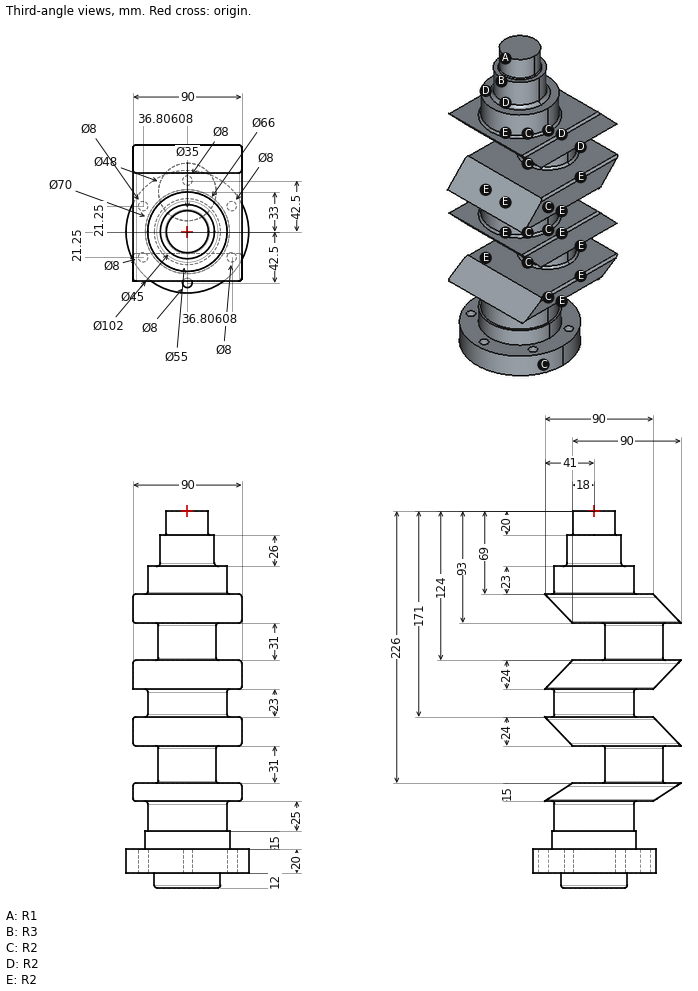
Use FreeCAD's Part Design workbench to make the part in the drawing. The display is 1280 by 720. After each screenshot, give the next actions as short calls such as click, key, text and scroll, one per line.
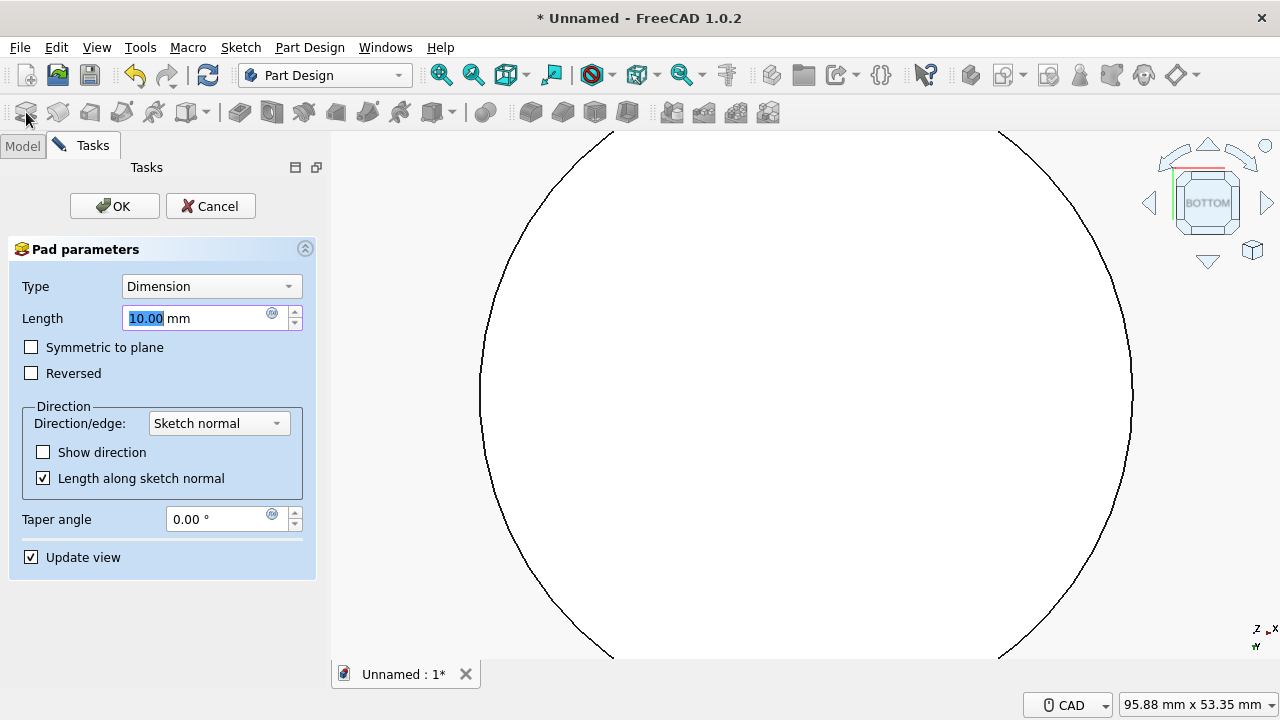
text(23)
key(Tab)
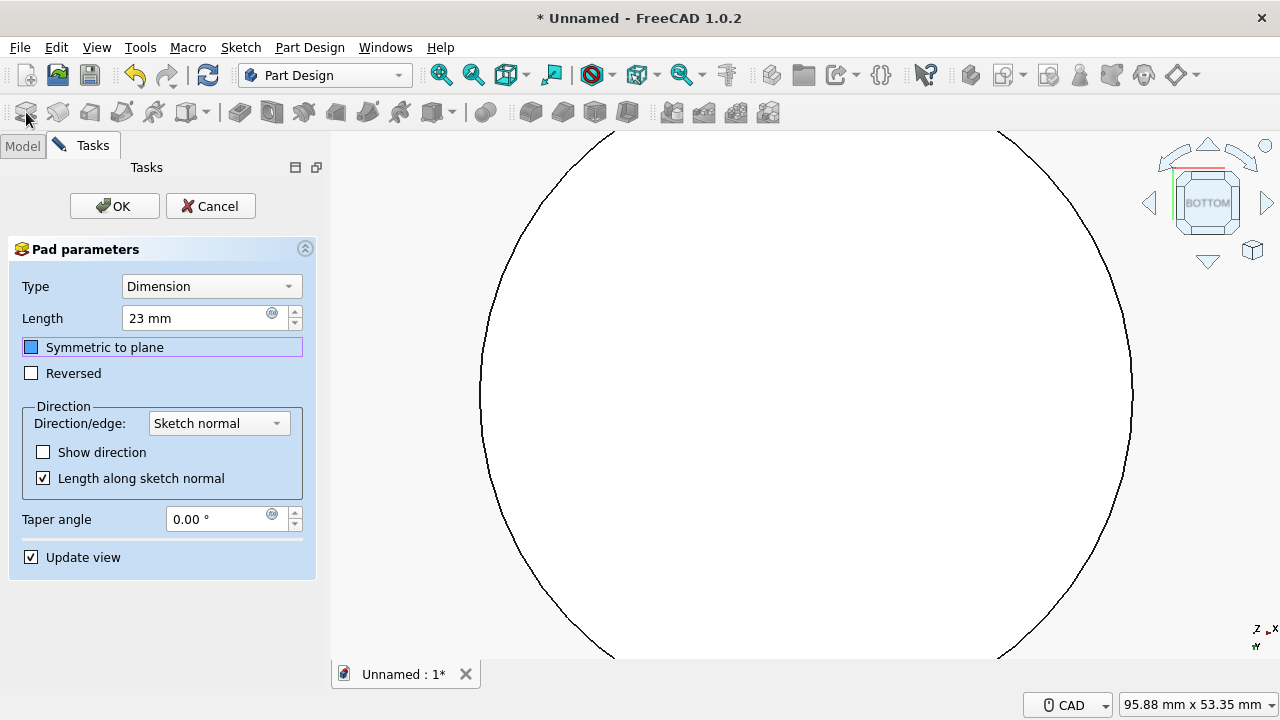
click(115, 206)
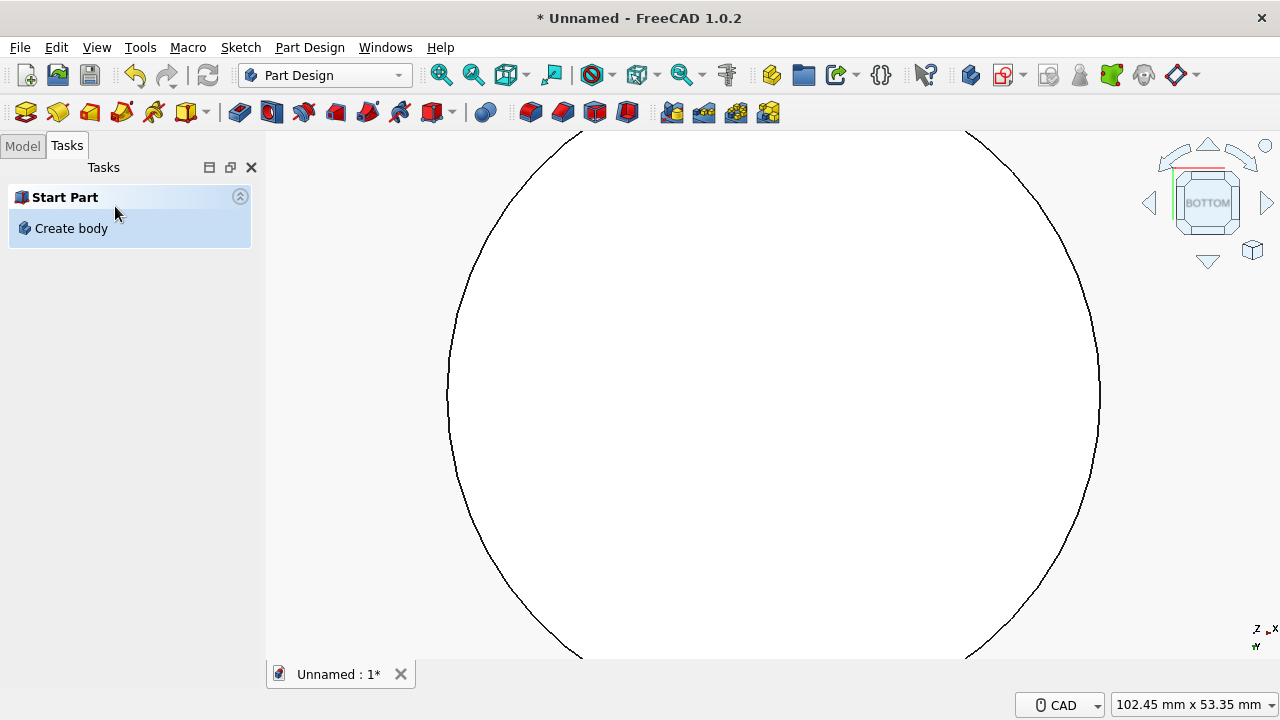
click(442, 76)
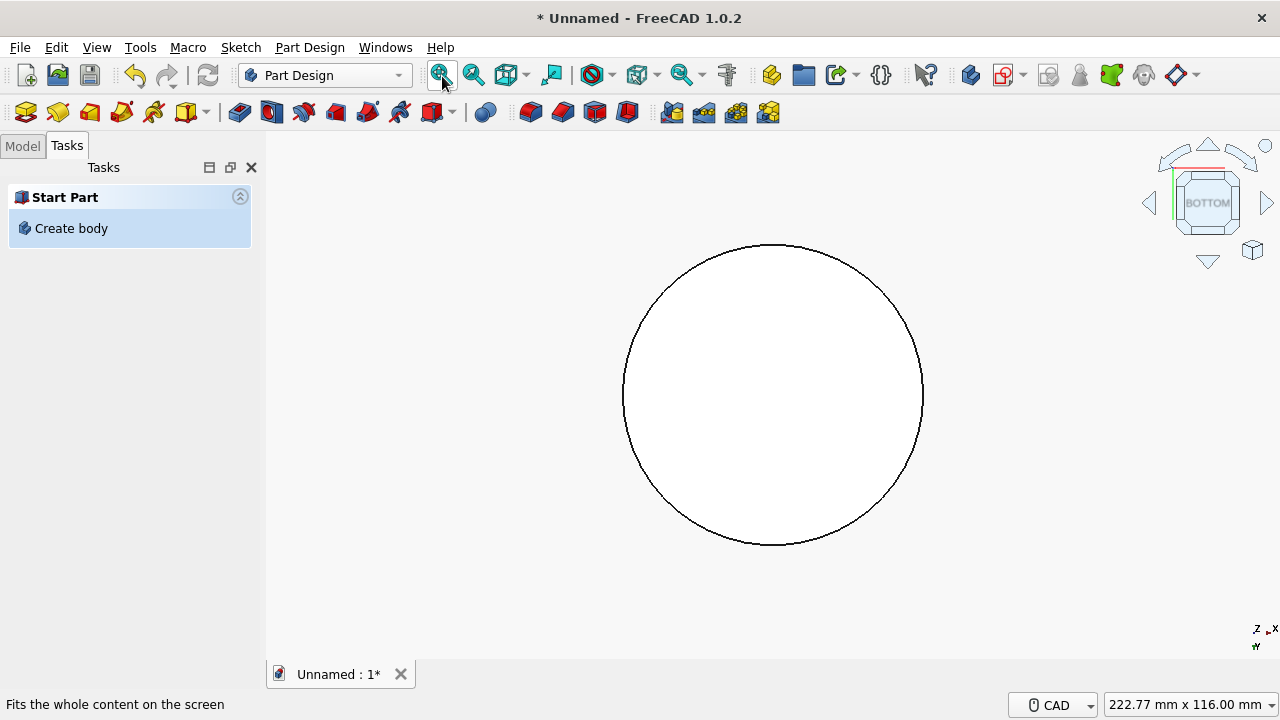
click(1004, 76)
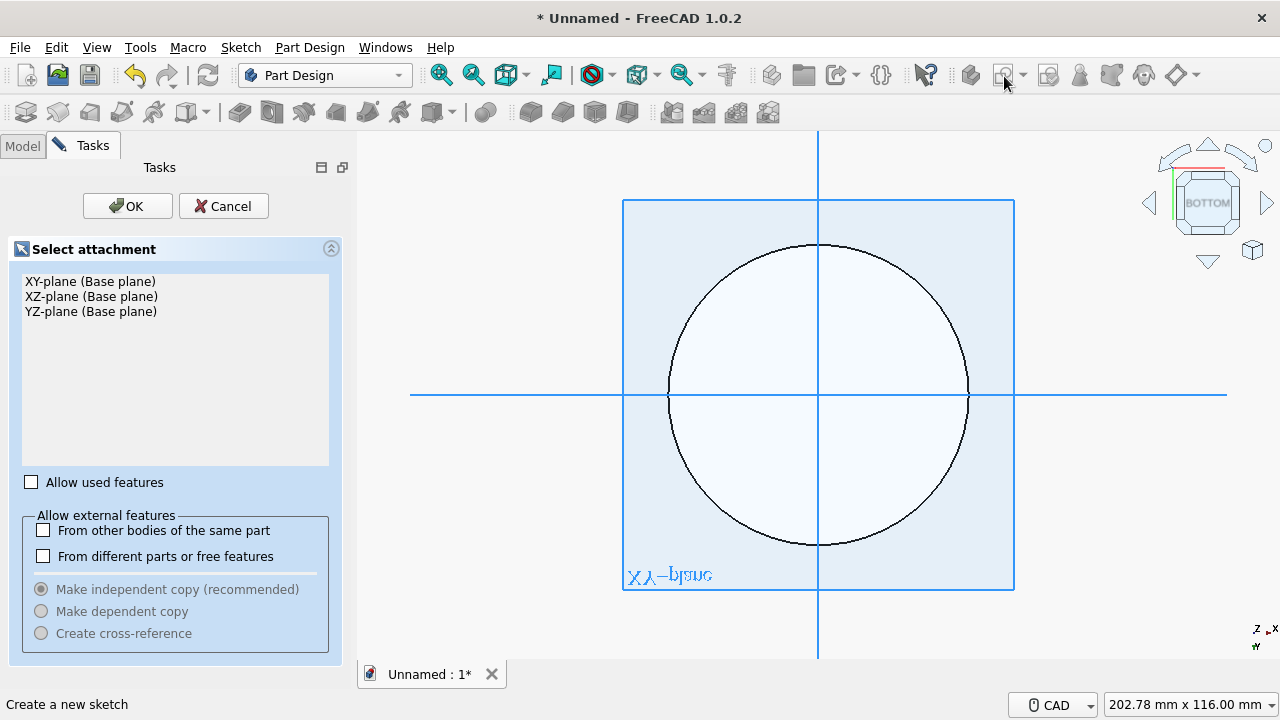
click(82, 312)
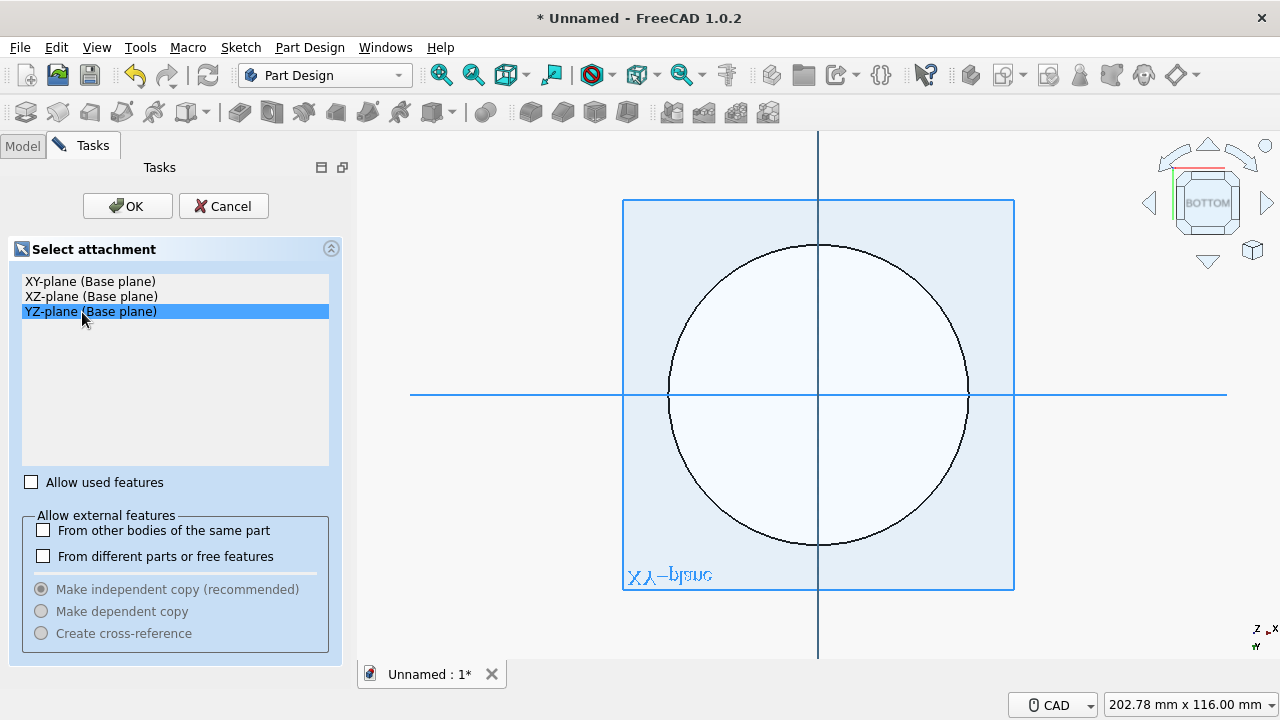
click(128, 206)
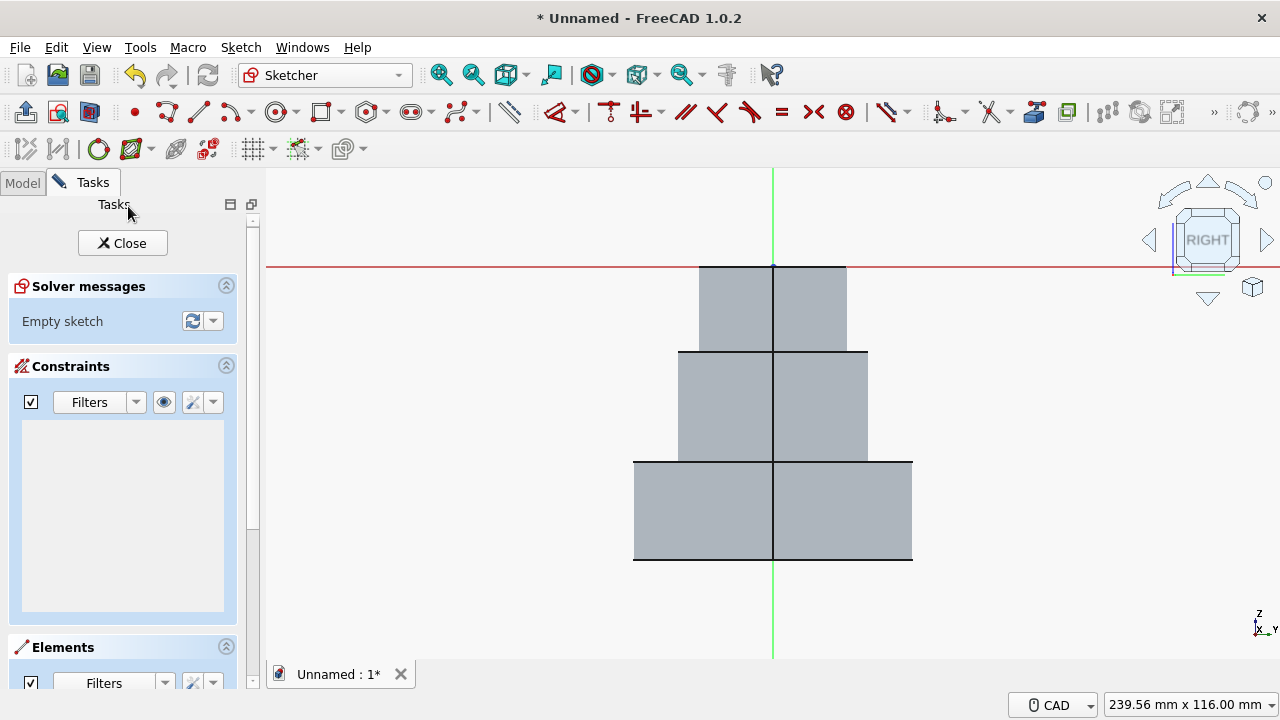
click(90, 112)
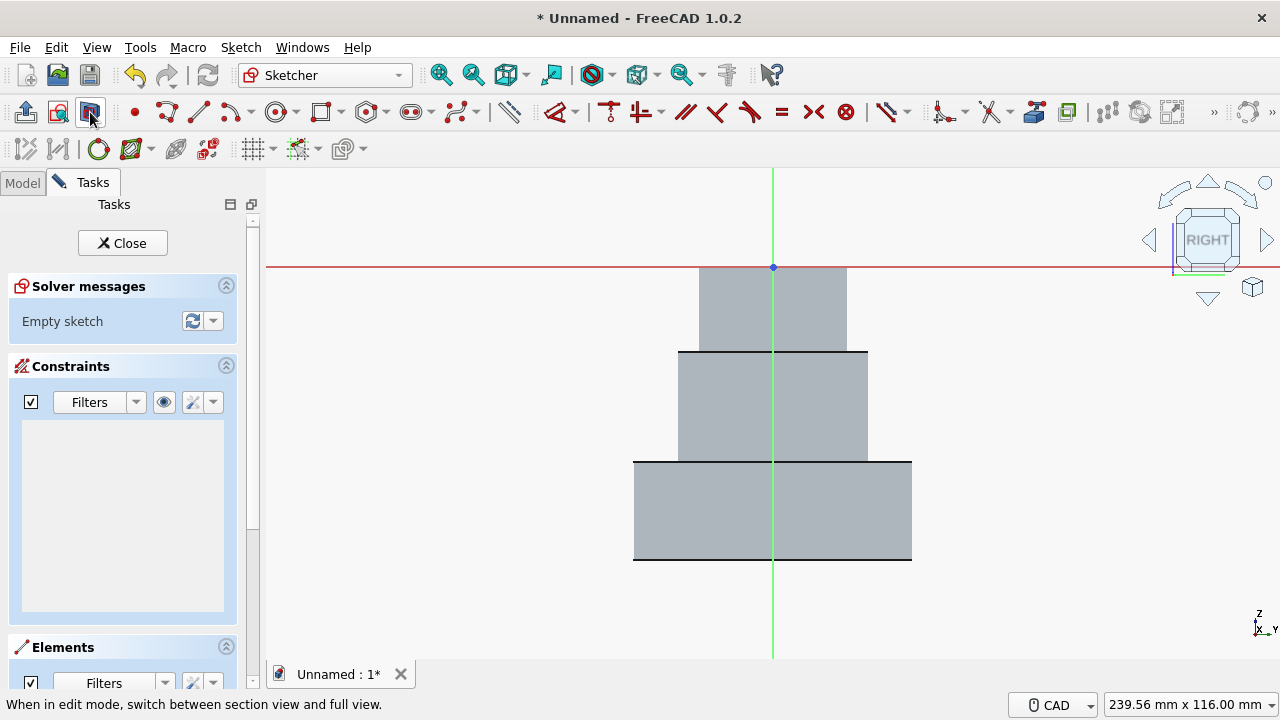
scroll(294, 196, down, 1)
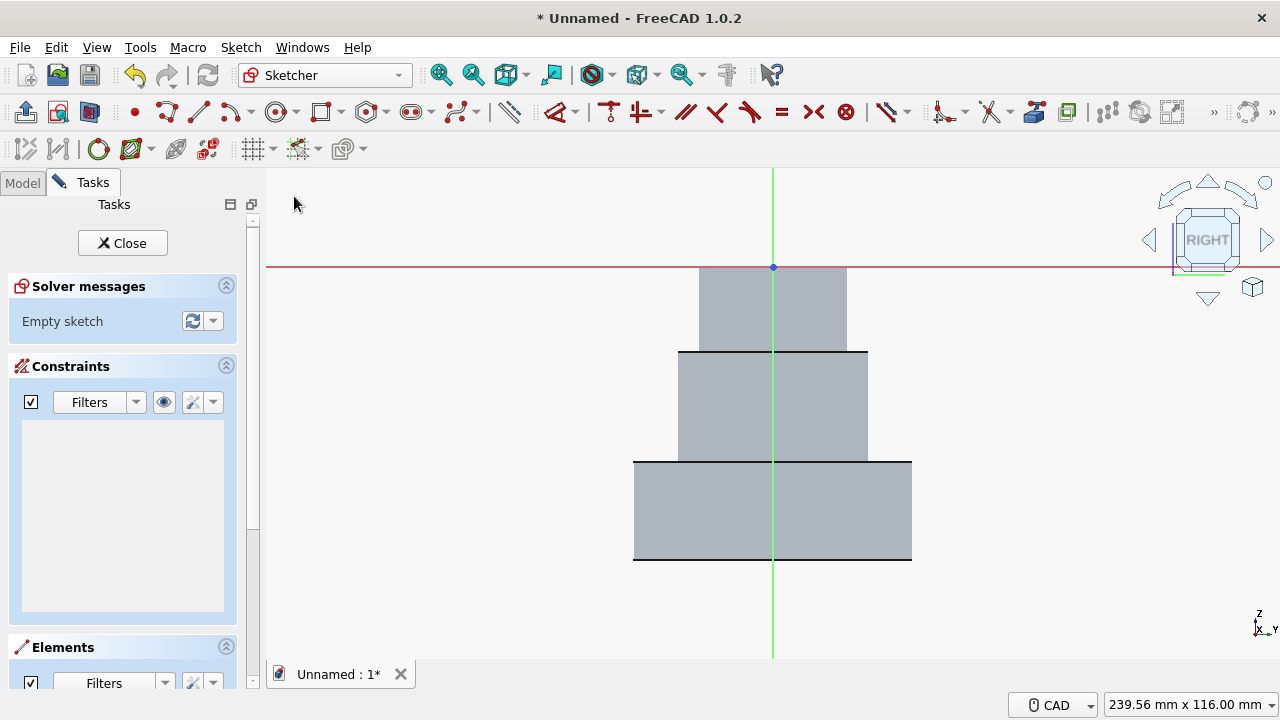
click(168, 112)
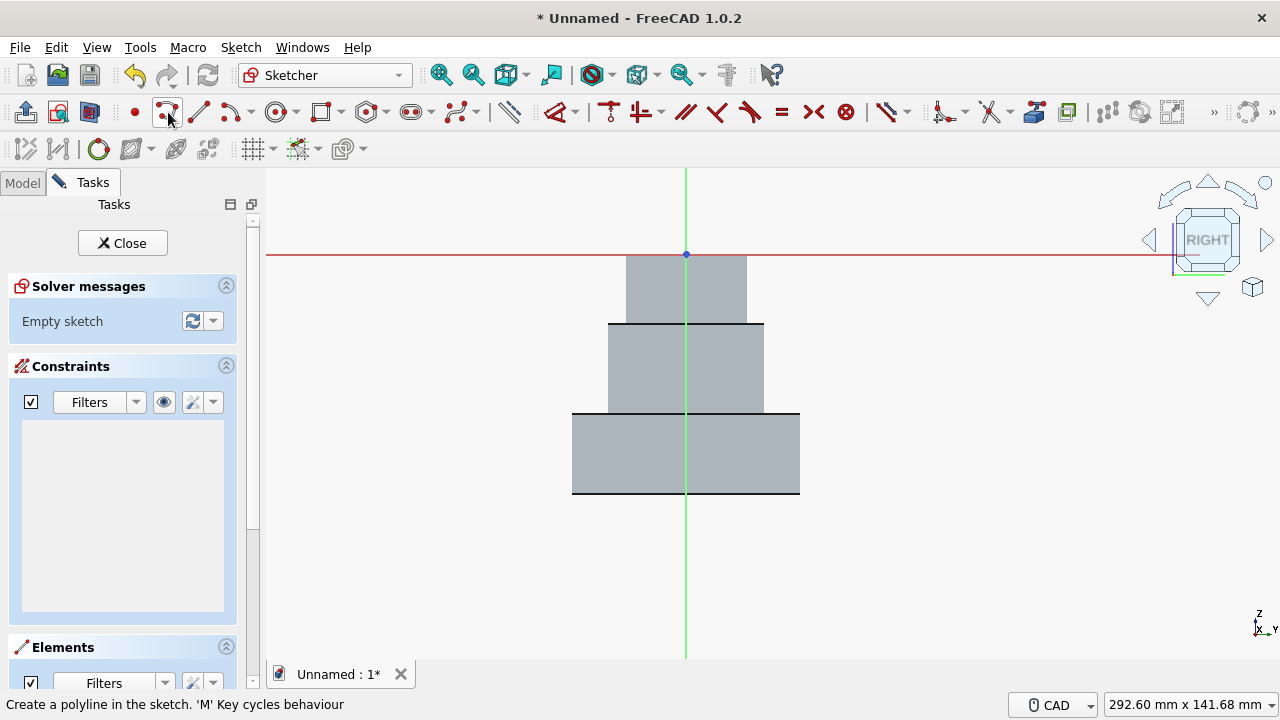
click(544, 494)
click(624, 577)
click(936, 577)
click(856, 494)
click(544, 495)
key(Escape)
key(Escape)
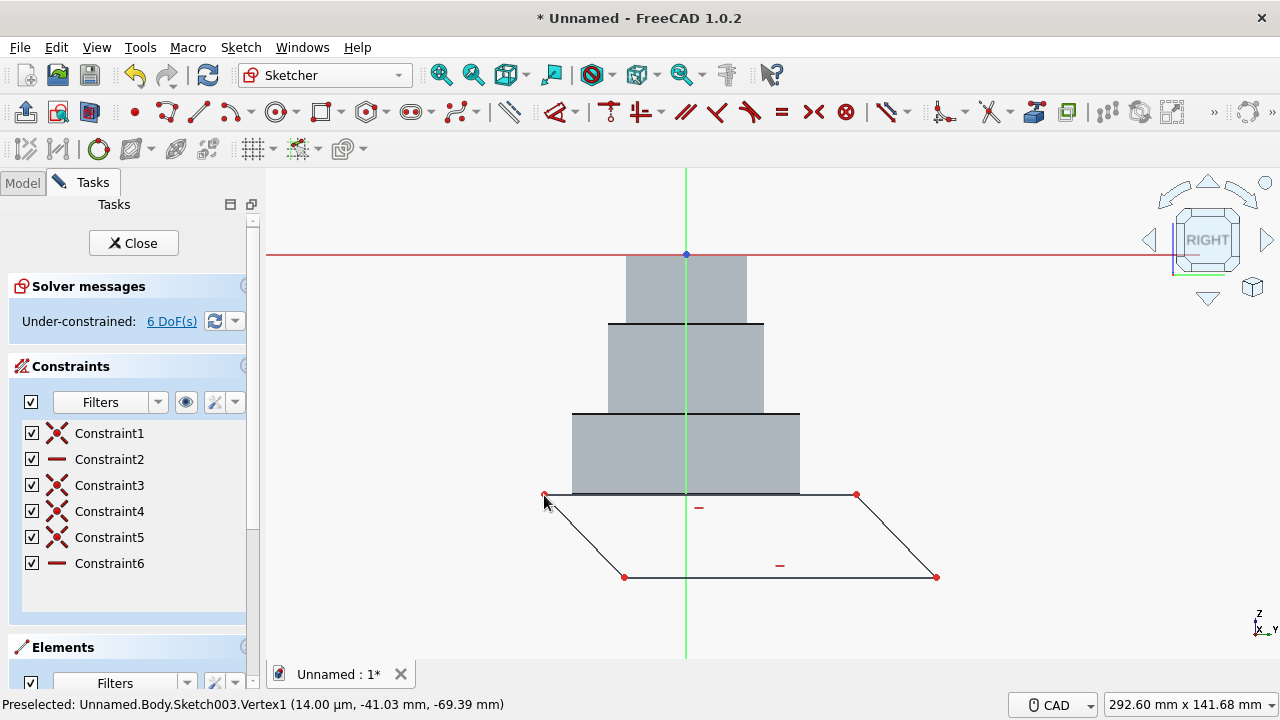
click(556, 112)